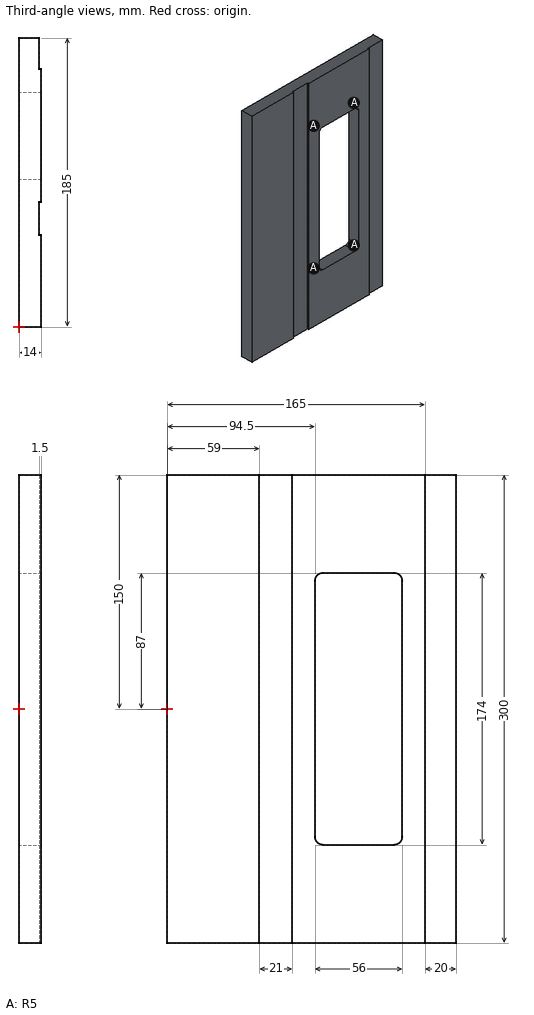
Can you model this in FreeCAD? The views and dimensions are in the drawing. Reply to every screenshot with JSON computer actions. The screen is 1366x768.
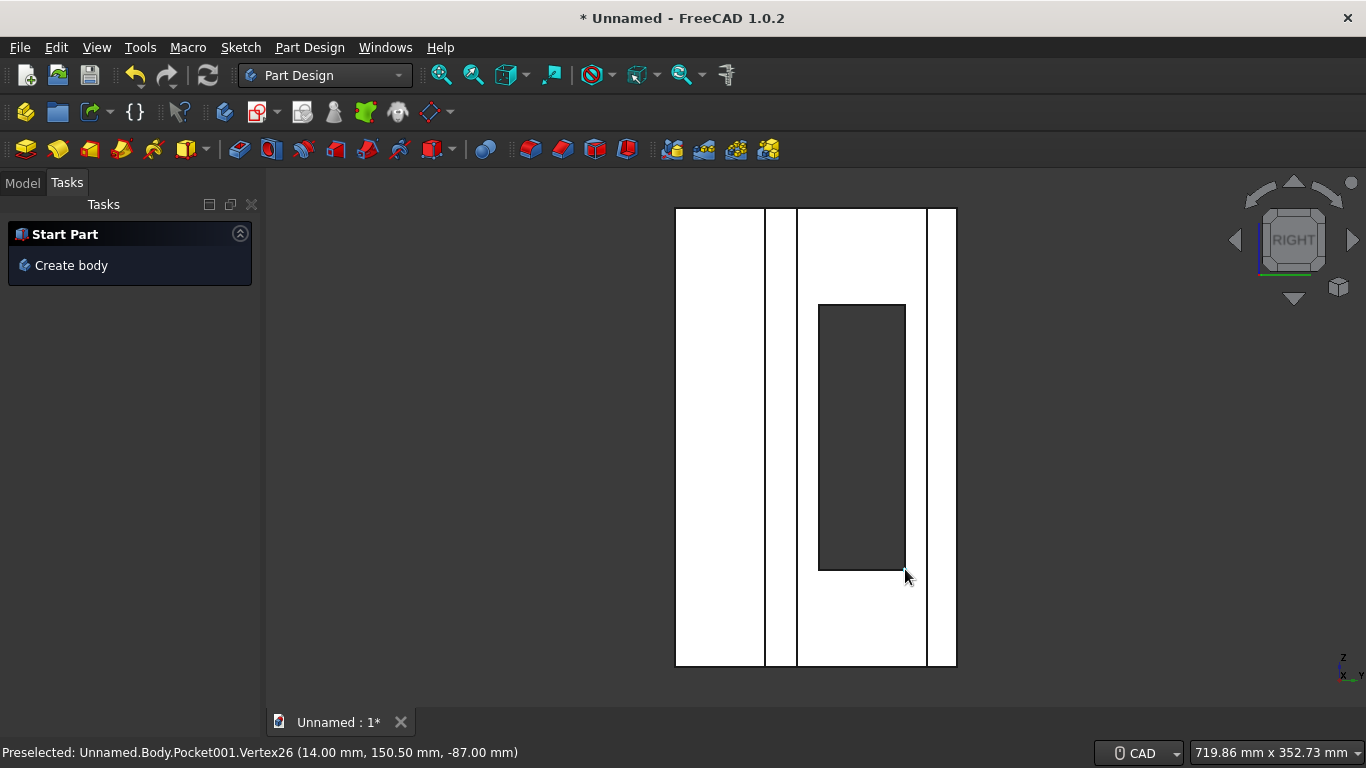
{"action": "key", "text": "5"}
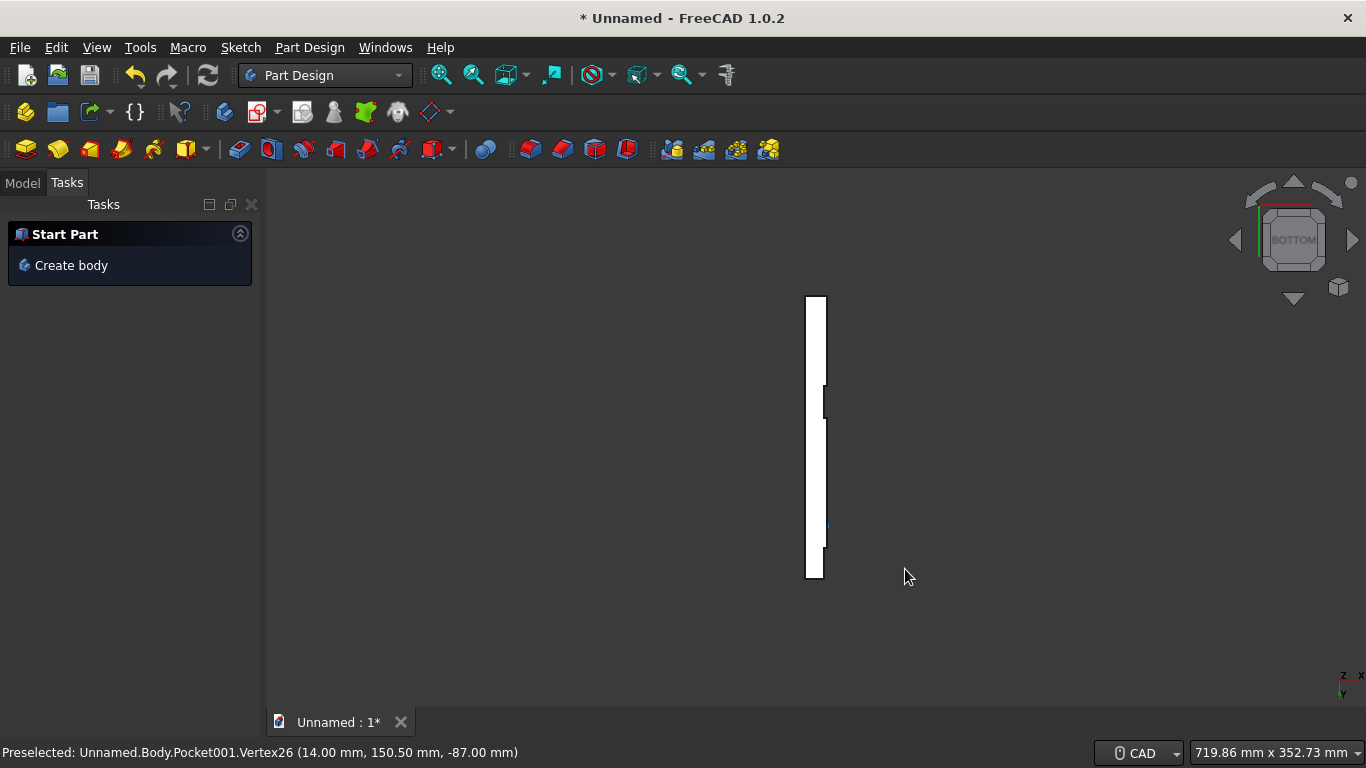
{"action": "scroll", "coordinate": [816, 525], "scroll_direction": "up", "scroll_amount": 4}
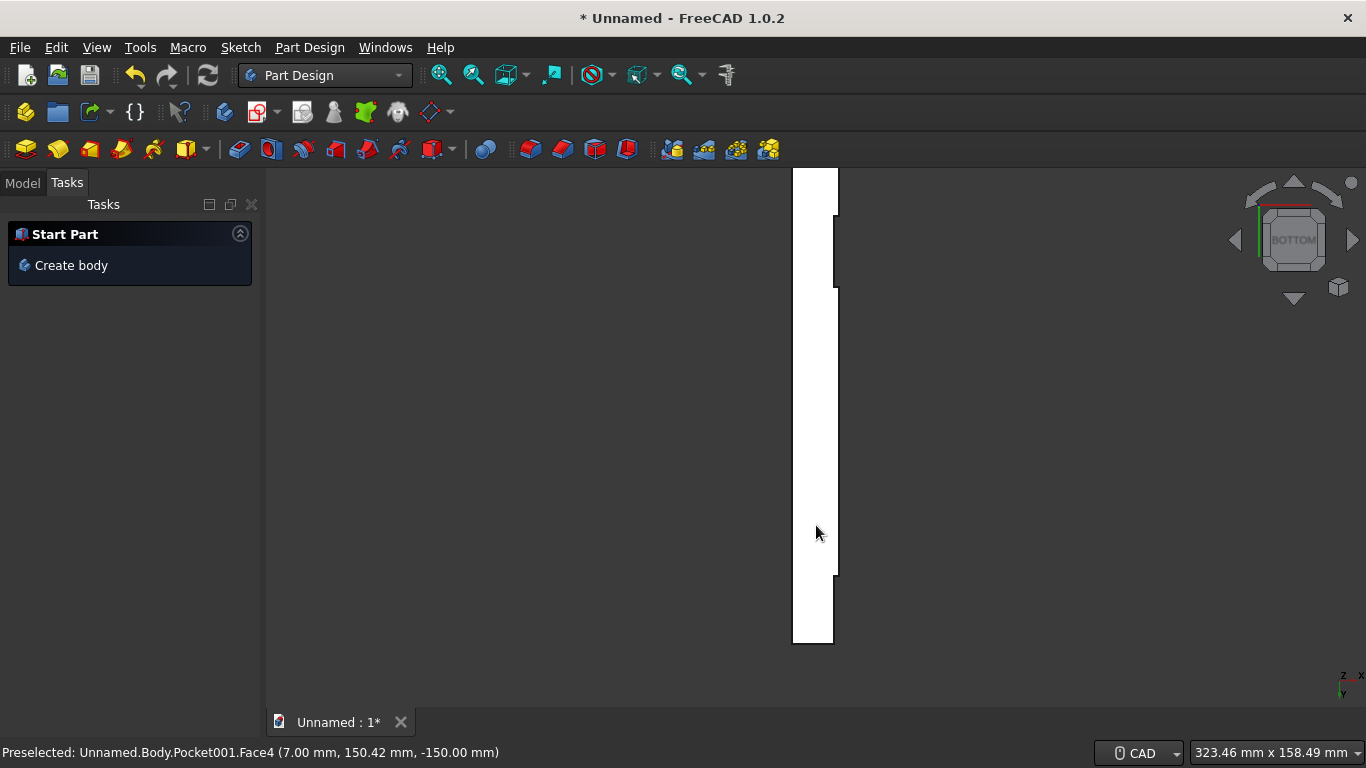
{"action": "left_click", "coordinate": [442, 76]}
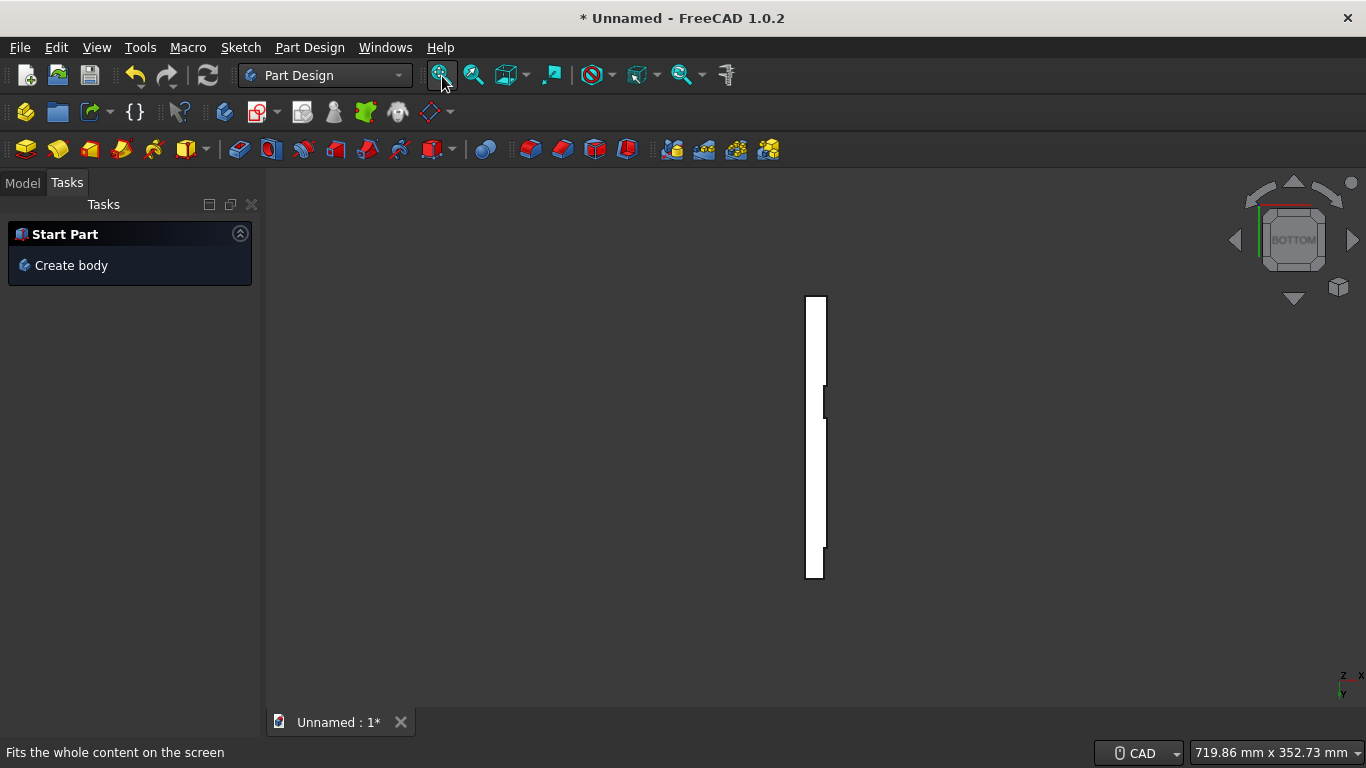
{"action": "key", "text": "4"}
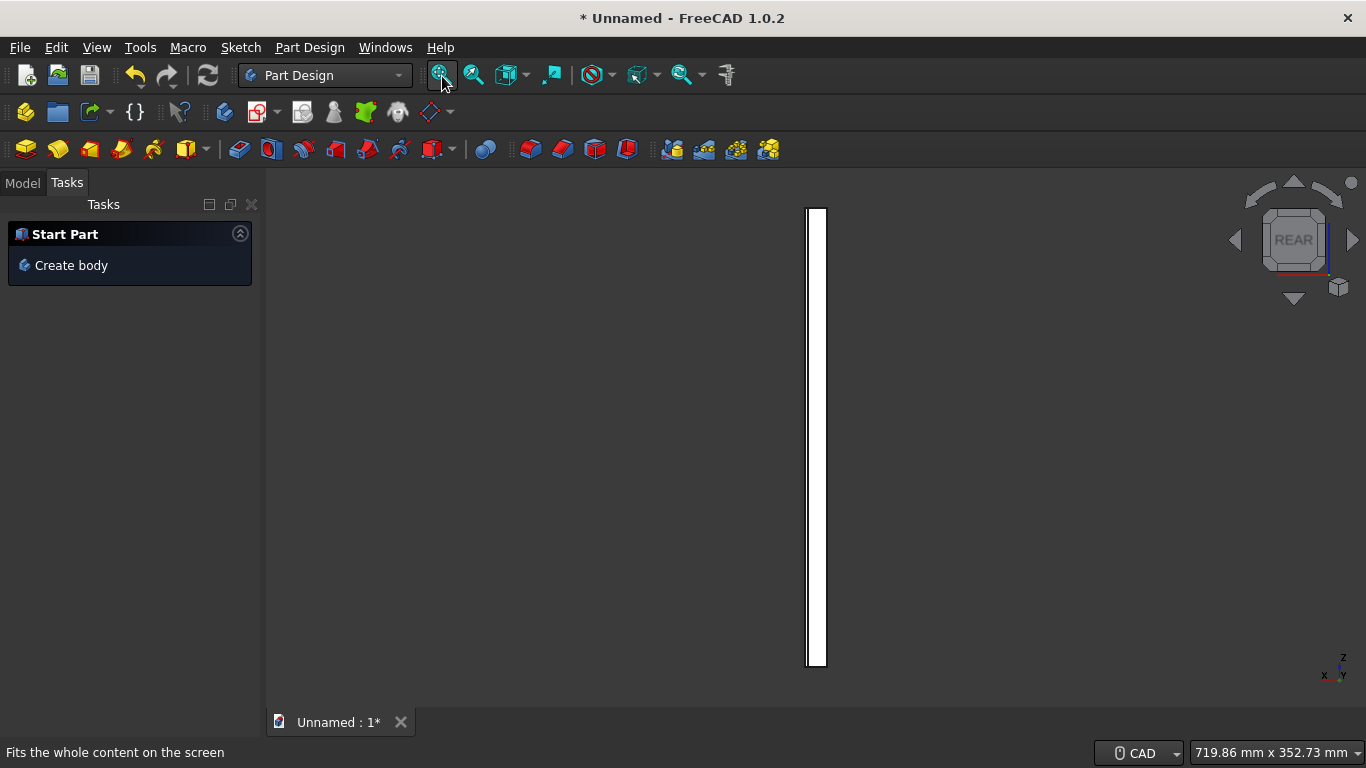
{"action": "scroll", "coordinate": [816, 569], "scroll_direction": "up", "scroll_amount": 4}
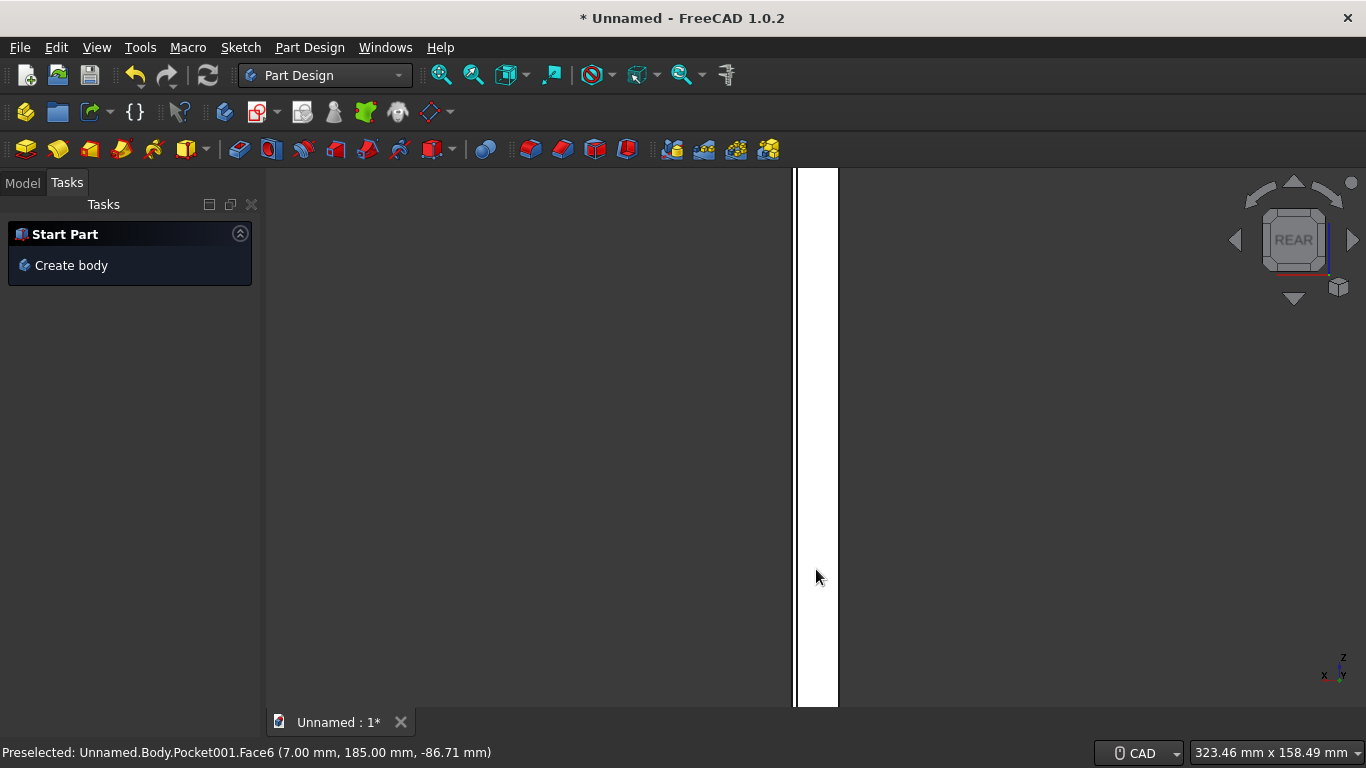
{"action": "left_click", "coordinate": [442, 76]}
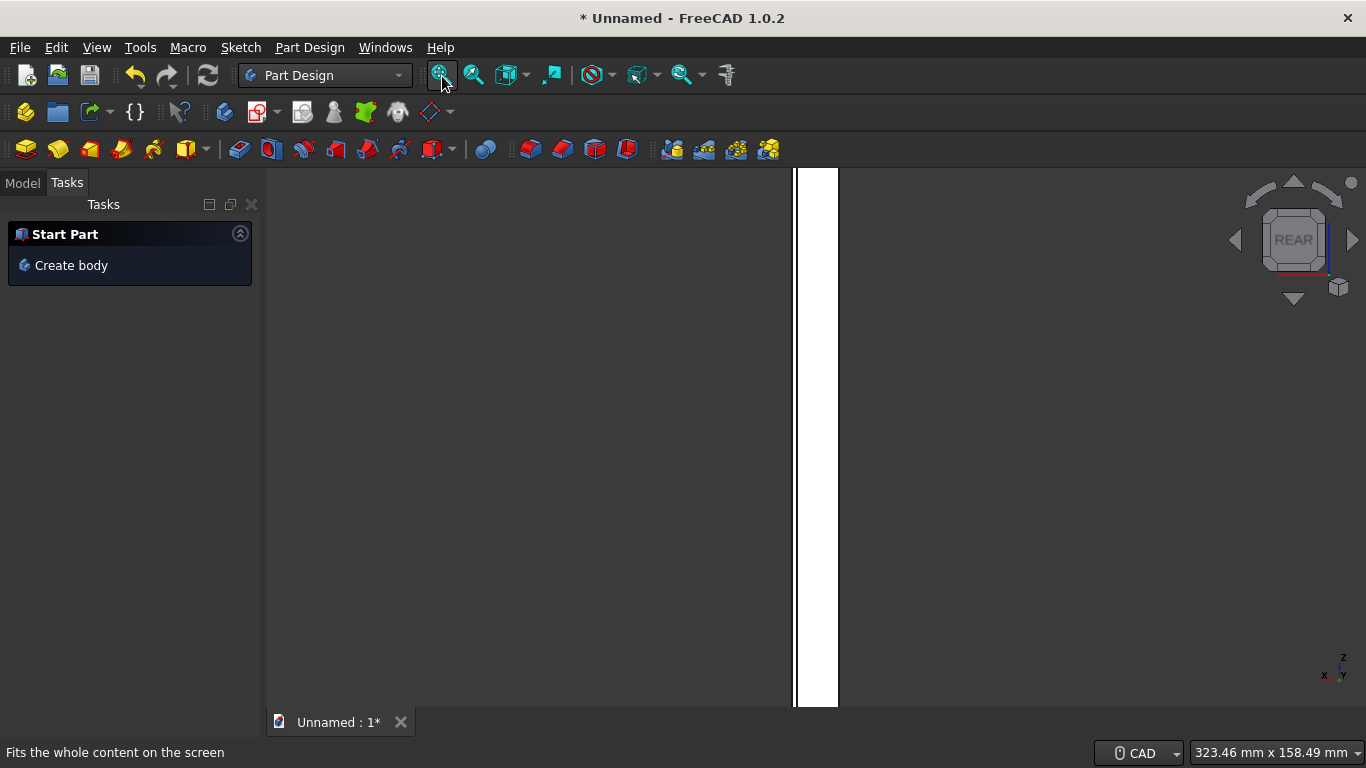
{"action": "key", "text": "6"}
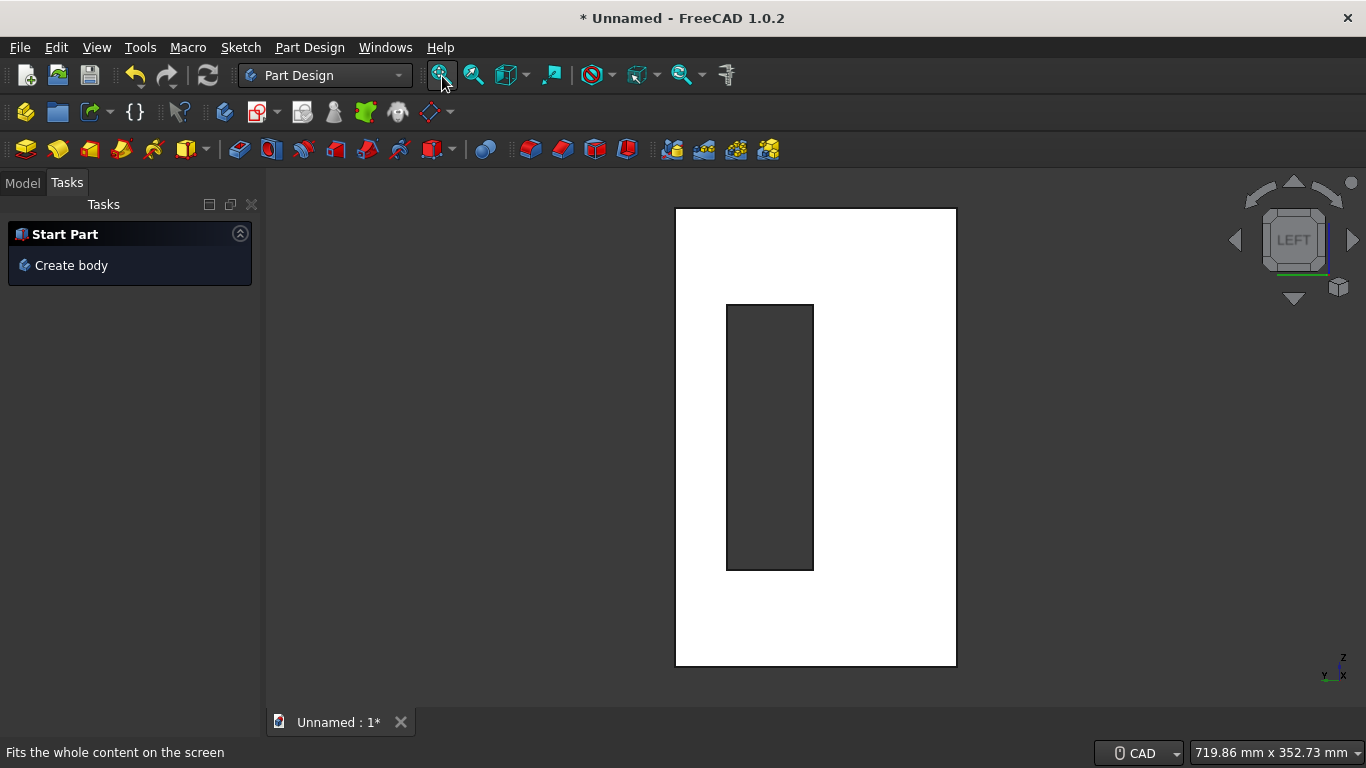
{"action": "scroll", "coordinate": [727, 569], "scroll_direction": "up", "scroll_amount": 4}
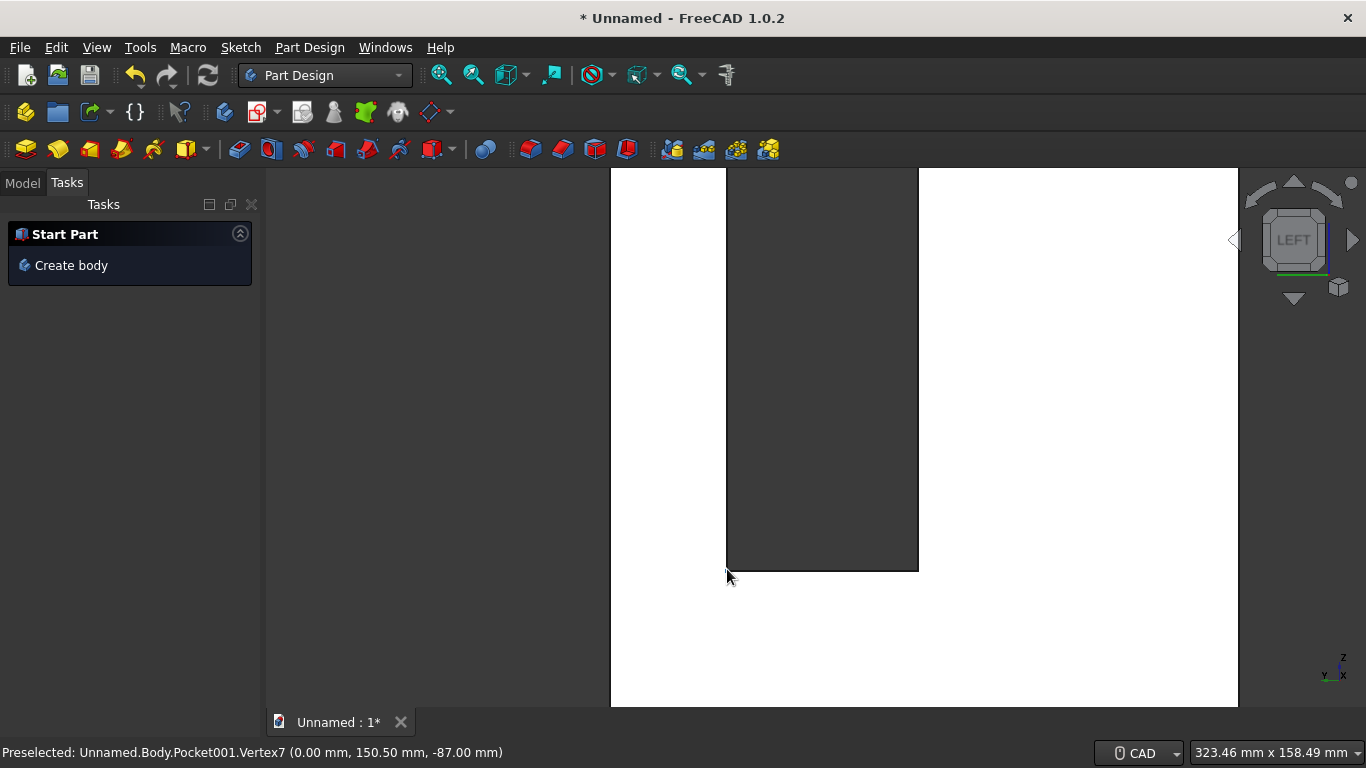
{"action": "left_click", "coordinate": [442, 76]}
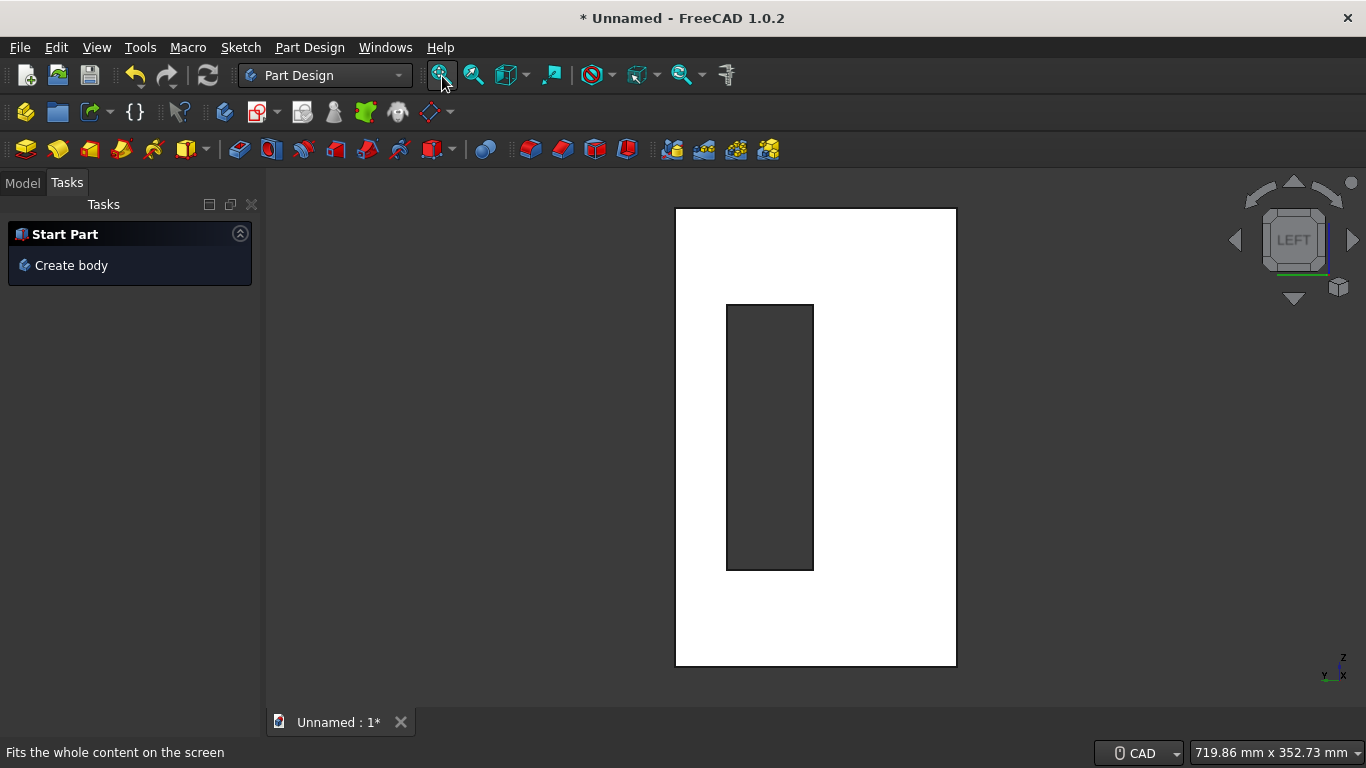
{"action": "key", "text": "v 3"}